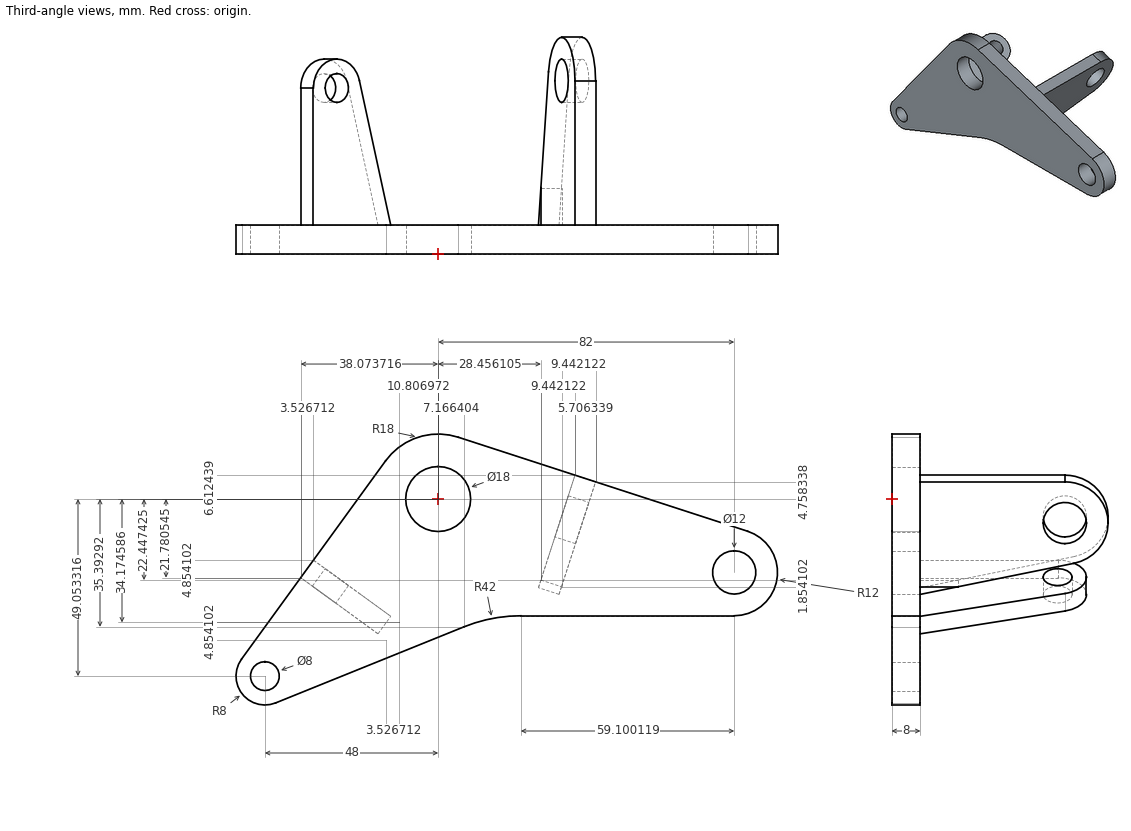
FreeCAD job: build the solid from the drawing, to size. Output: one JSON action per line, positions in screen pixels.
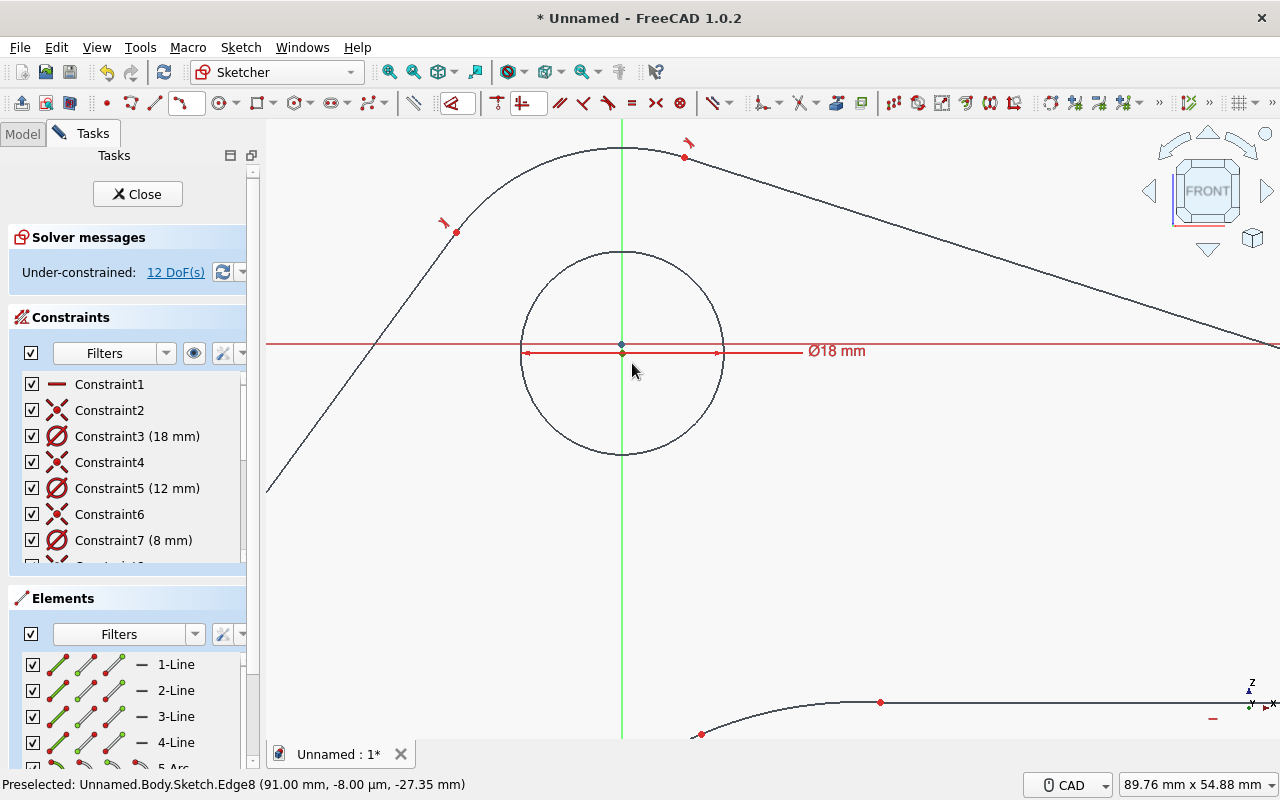
{"action": "key", "text": "c"}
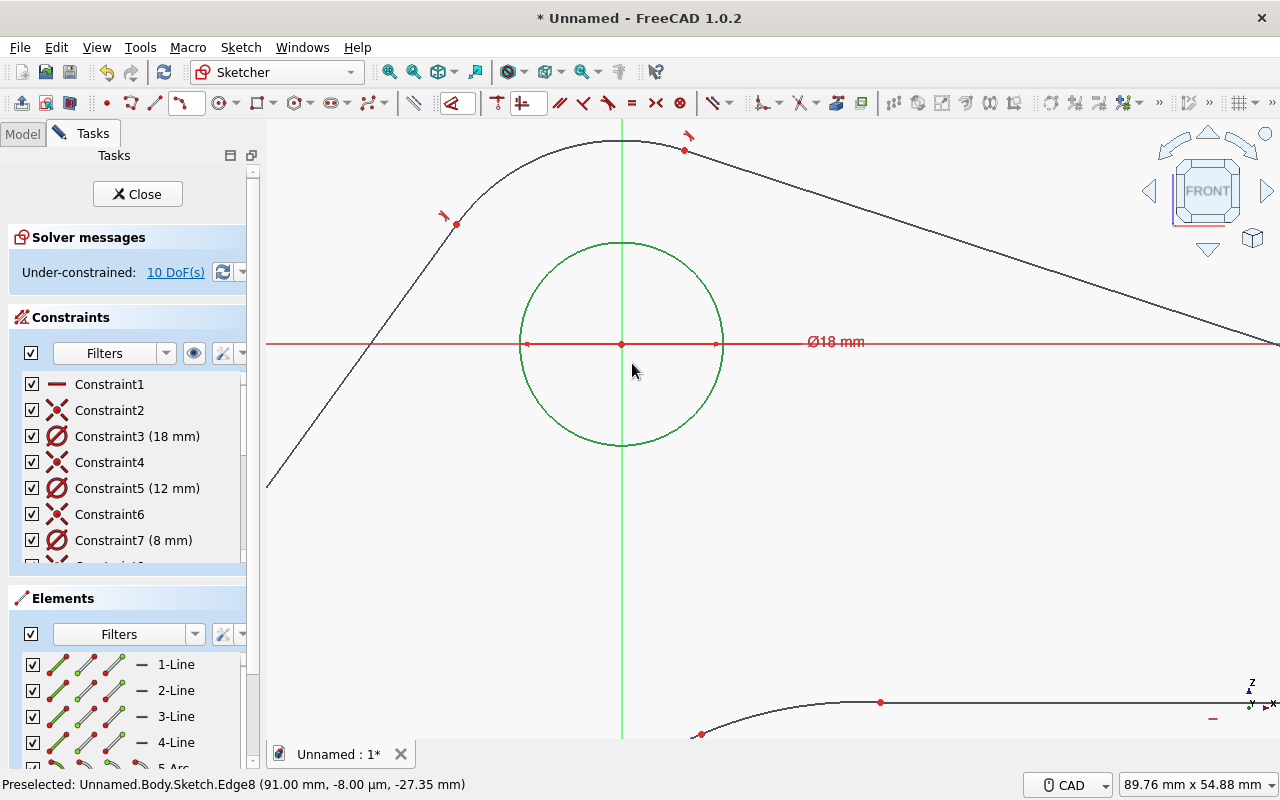
{"action": "left_click", "coordinate": [452, 104]}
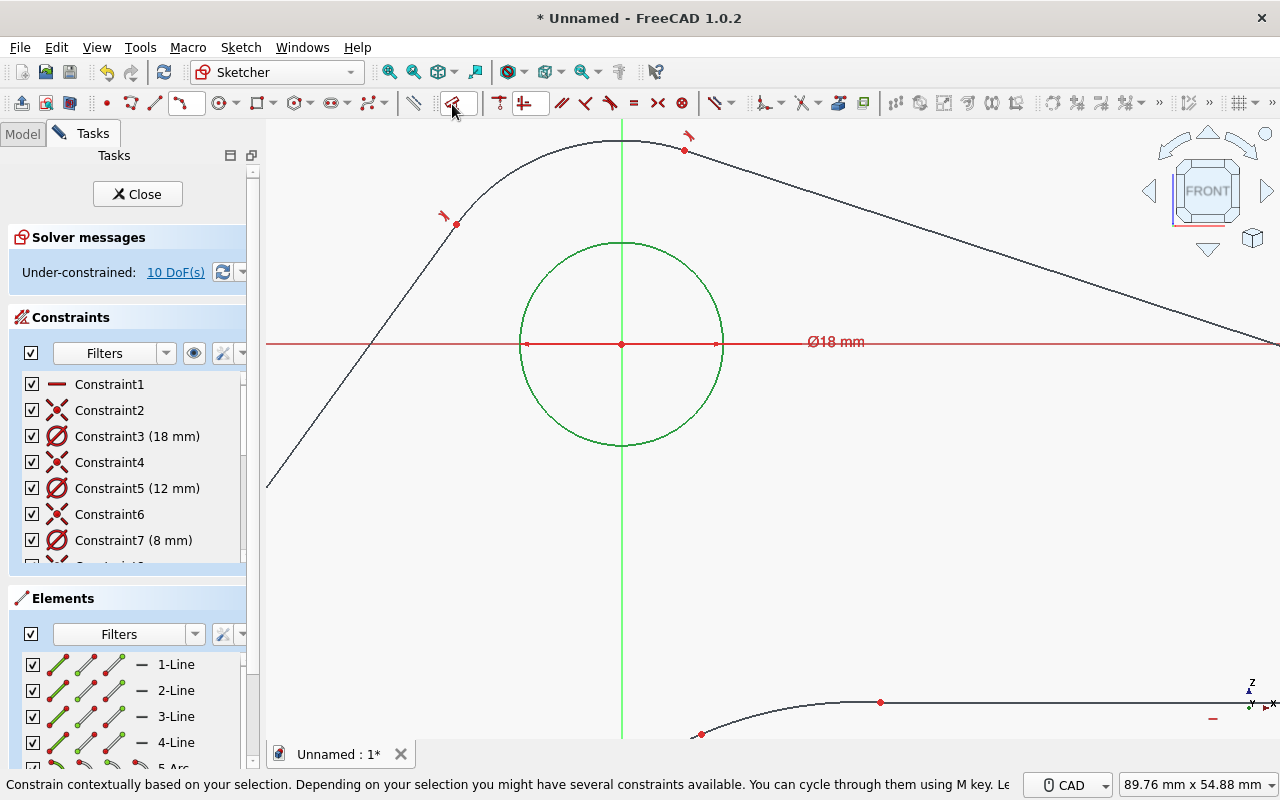
{"action": "left_click", "coordinate": [826, 703]}
{"action": "left_click", "coordinate": [823, 671]}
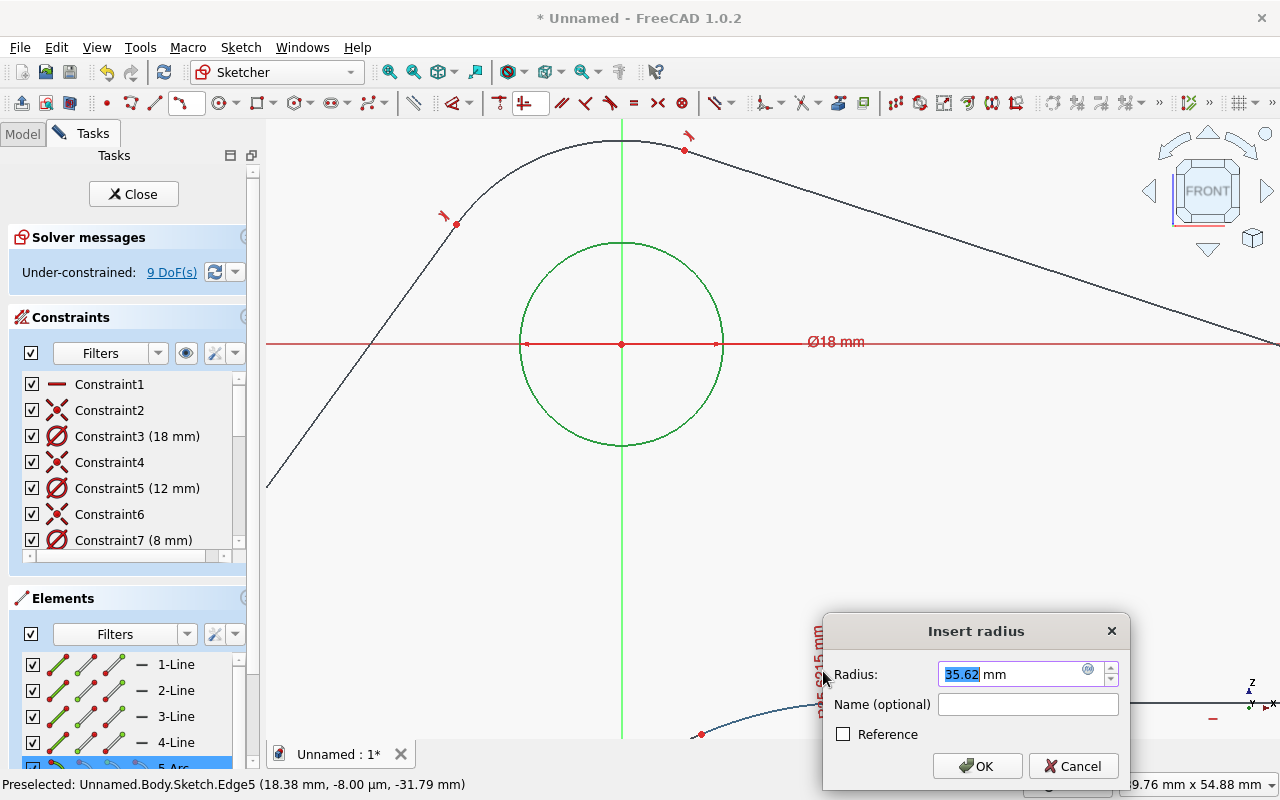
{"action": "type", "text": "42"}
{"action": "key", "text": "Return"}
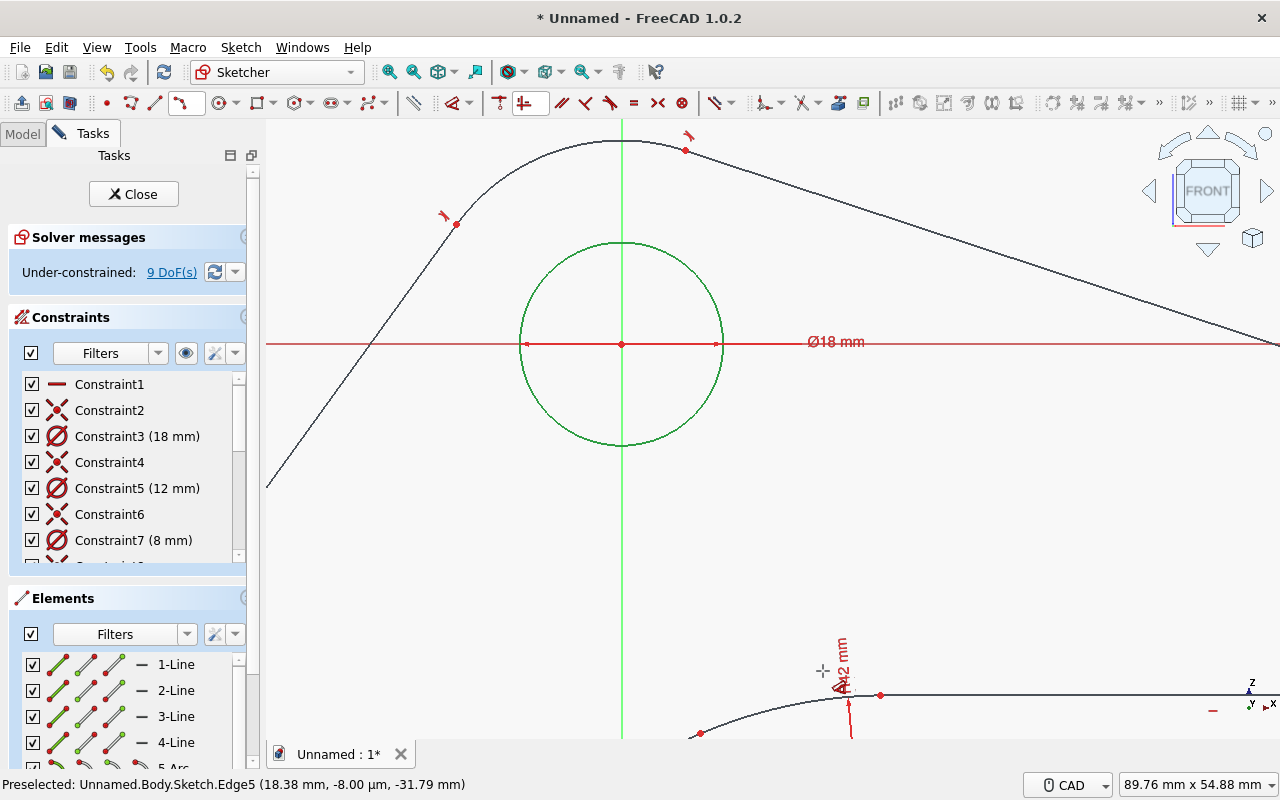
{"action": "scroll", "coordinate": [623, 349], "scroll_direction": "down", "scroll_amount": 5}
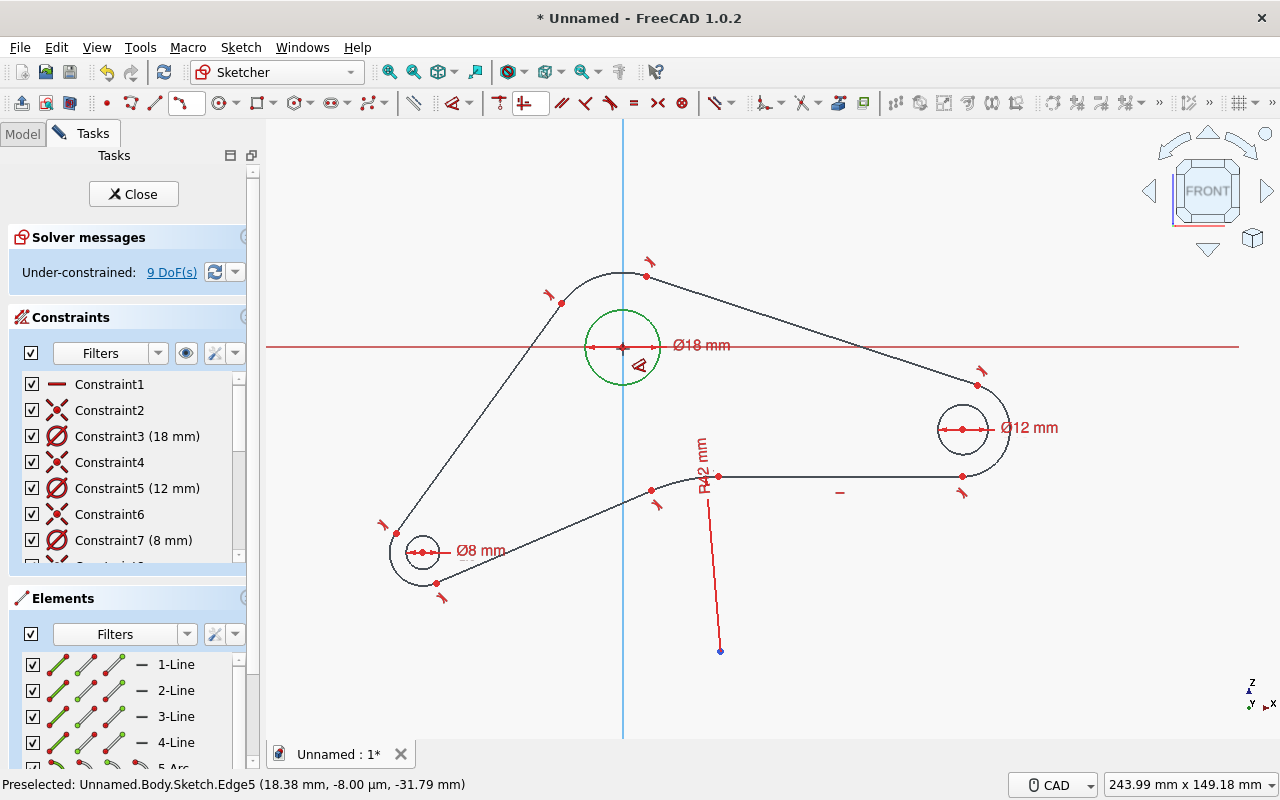
{"action": "left_click", "coordinate": [390, 558]}
{"action": "left_click", "coordinate": [358, 563]}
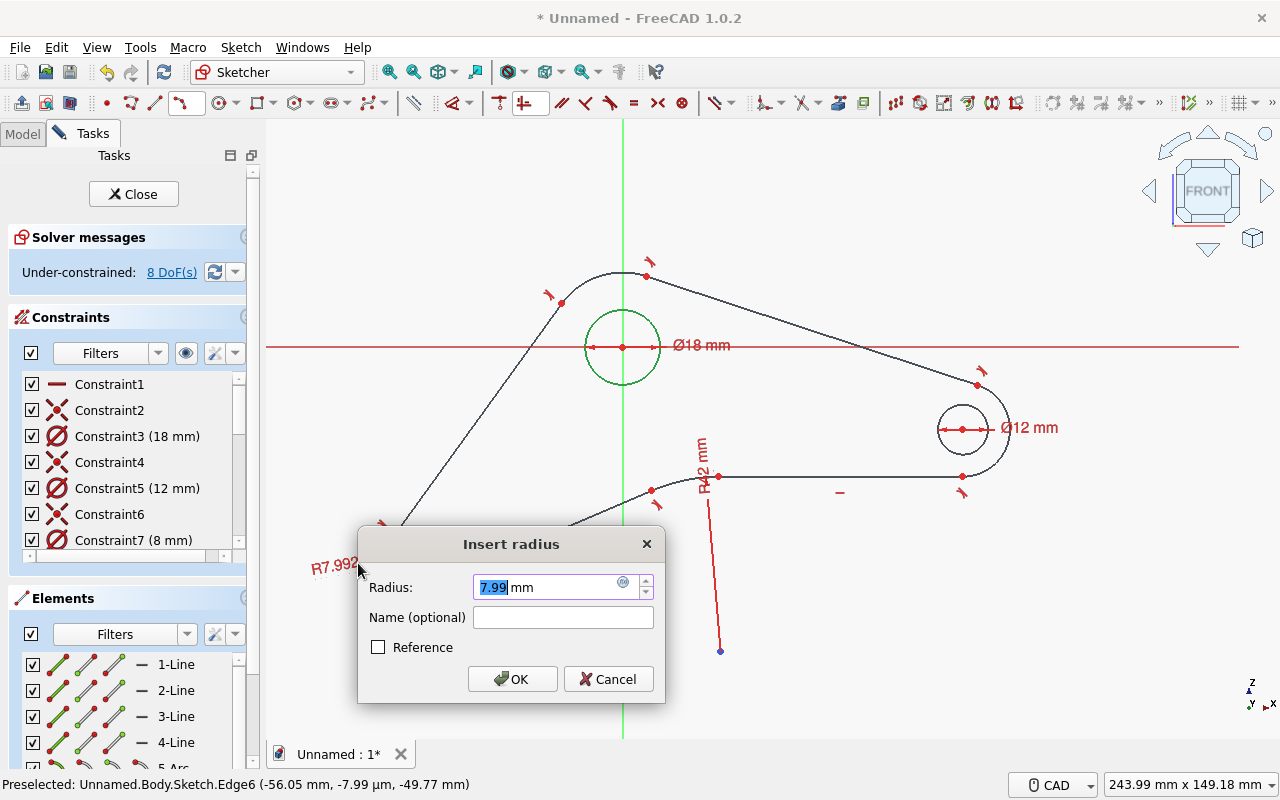
{"action": "type", "text": "8"}
{"action": "key", "text": "Return"}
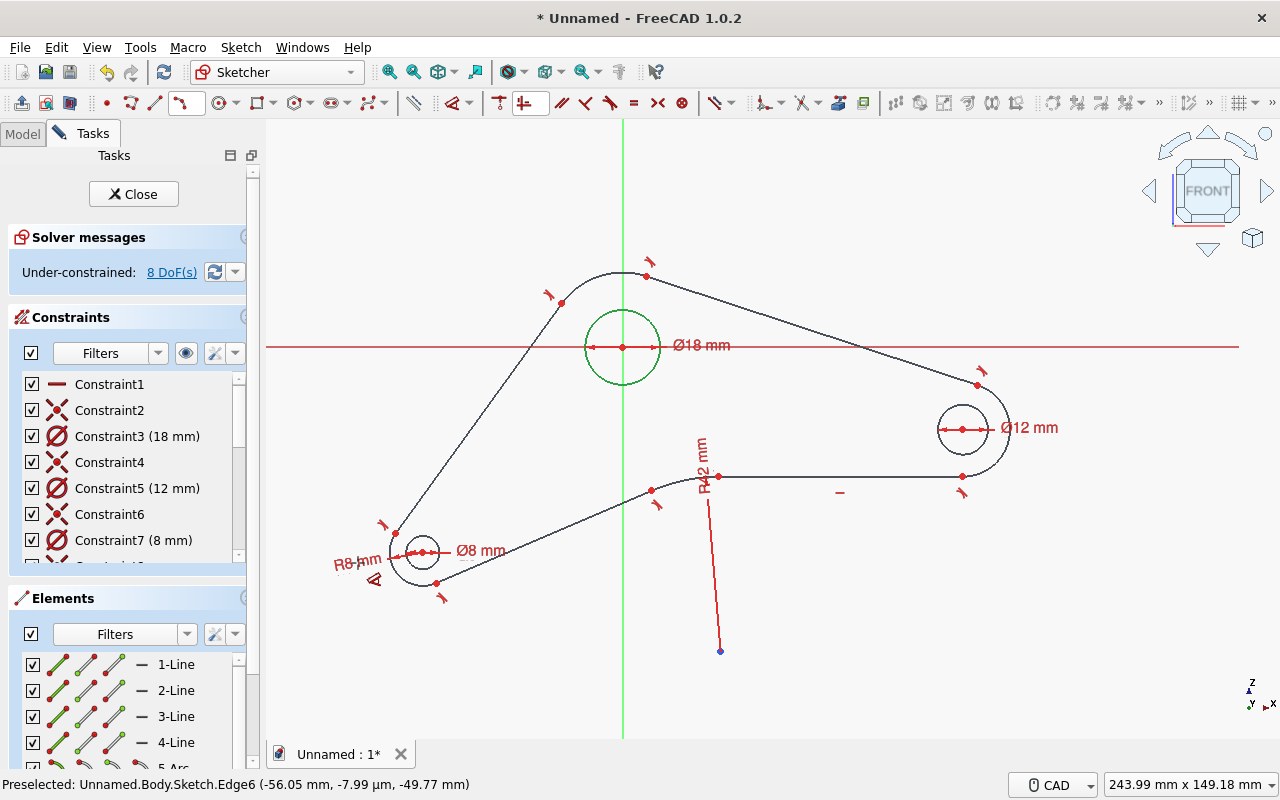
{"action": "left_click", "coordinate": [583, 284]}
{"action": "left_click", "coordinate": [566, 257]}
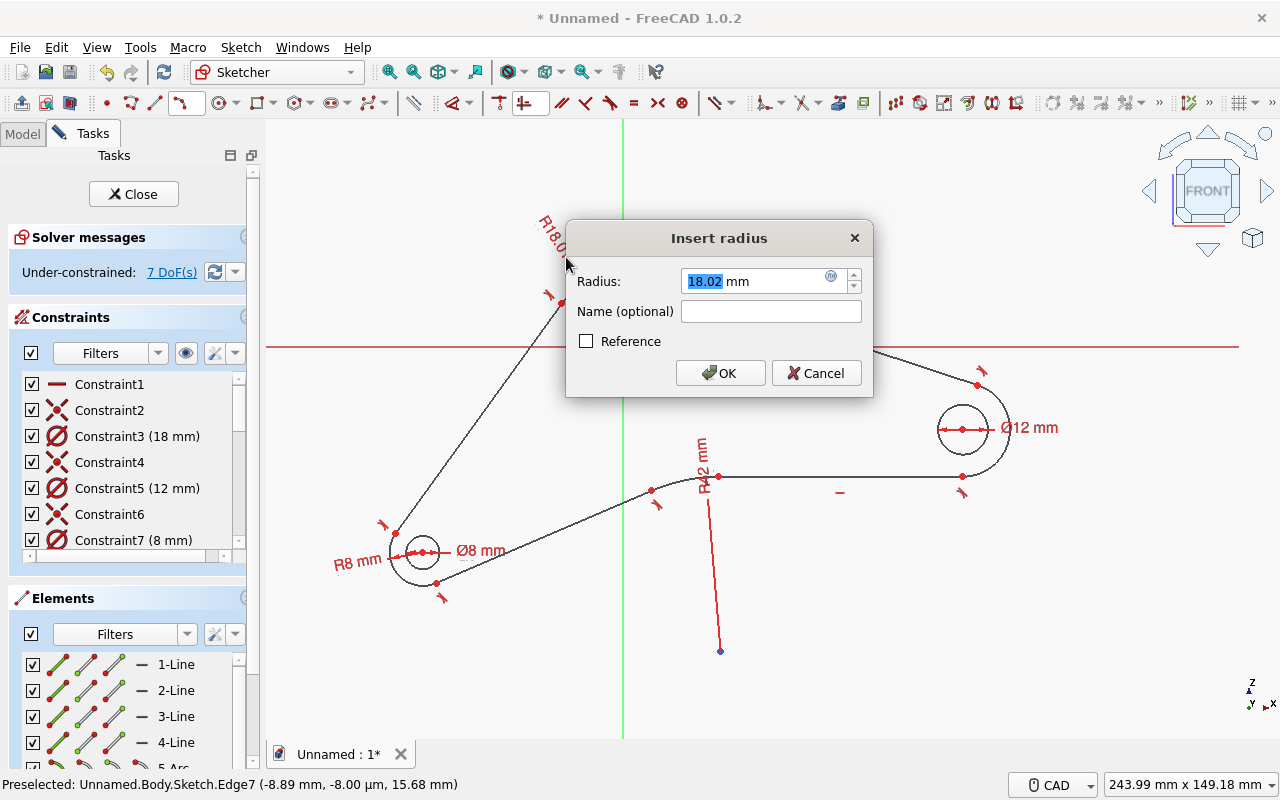
{"action": "type", "text": "18"}
{"action": "key", "text": "Return"}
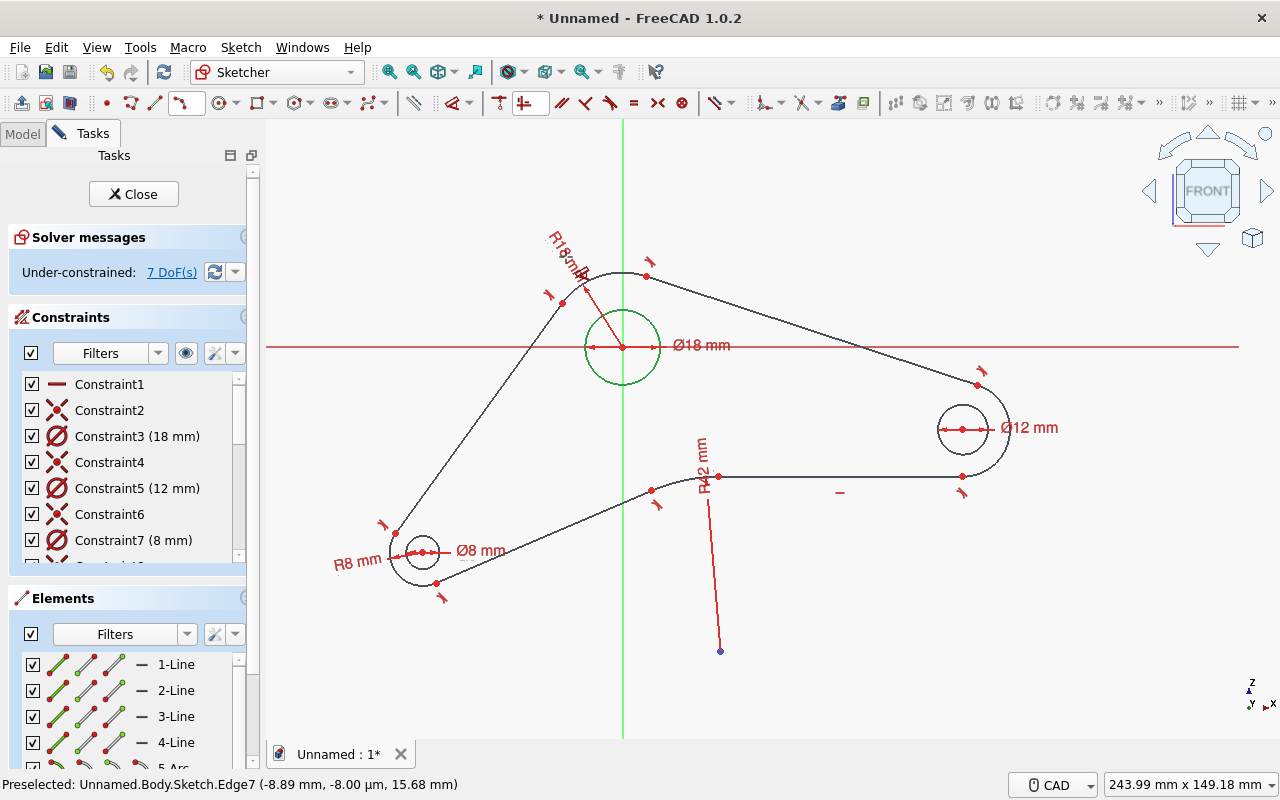
{"action": "left_click", "coordinate": [998, 461]}
{"action": "left_click", "coordinate": [1022, 482]}